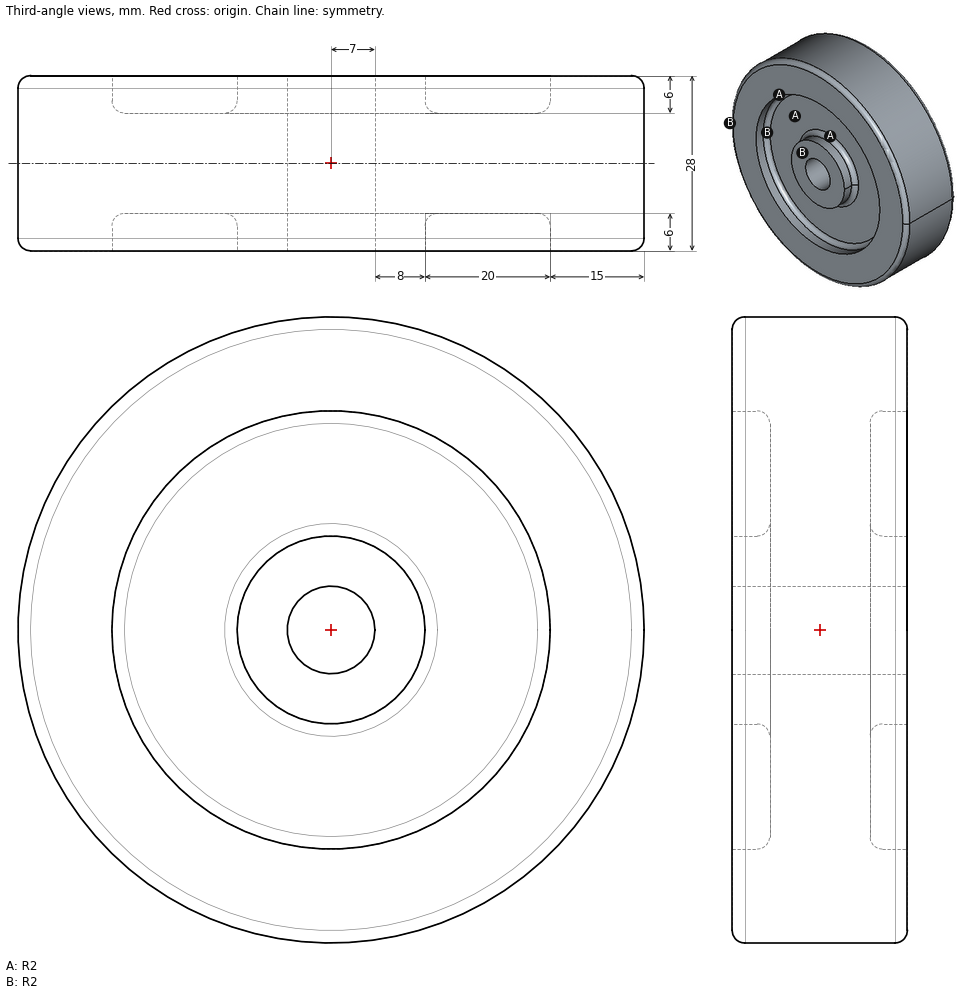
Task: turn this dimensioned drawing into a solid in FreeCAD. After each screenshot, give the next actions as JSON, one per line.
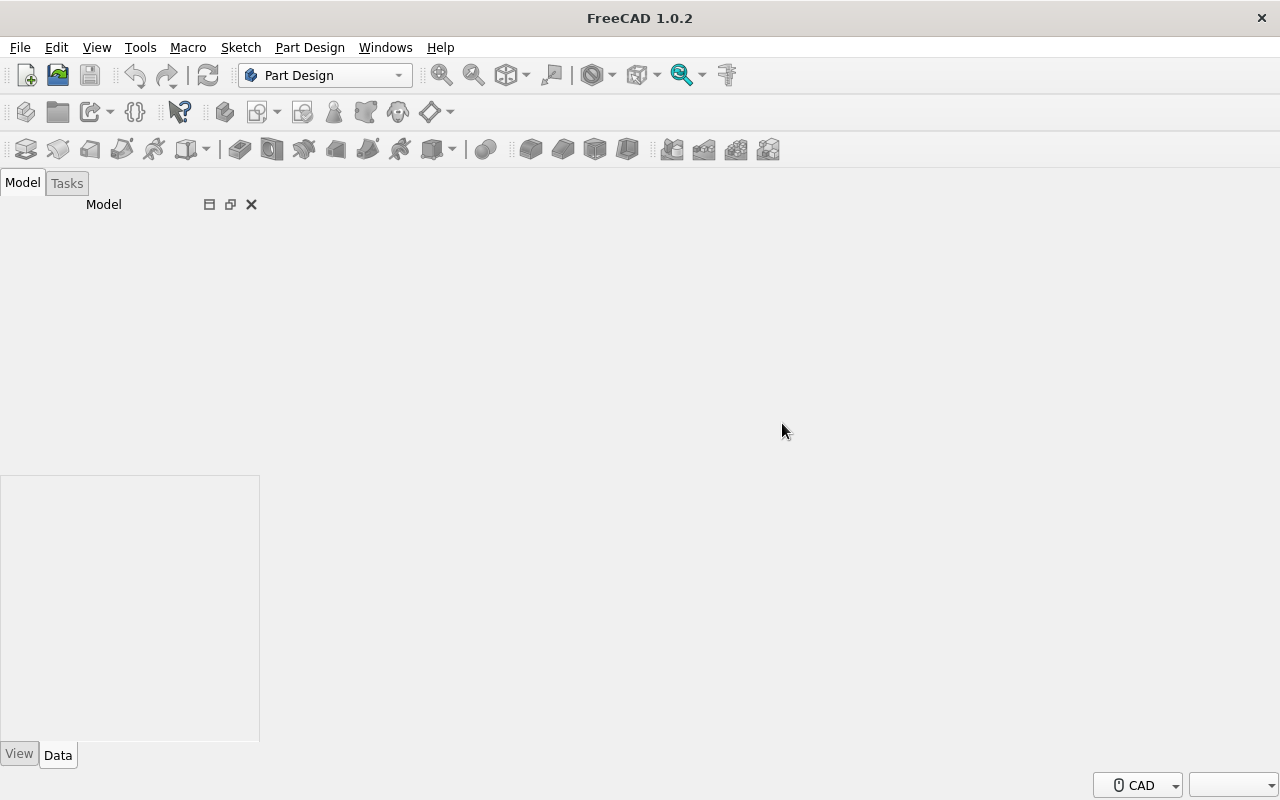
{"action": "left_click", "coordinate": [26, 76]}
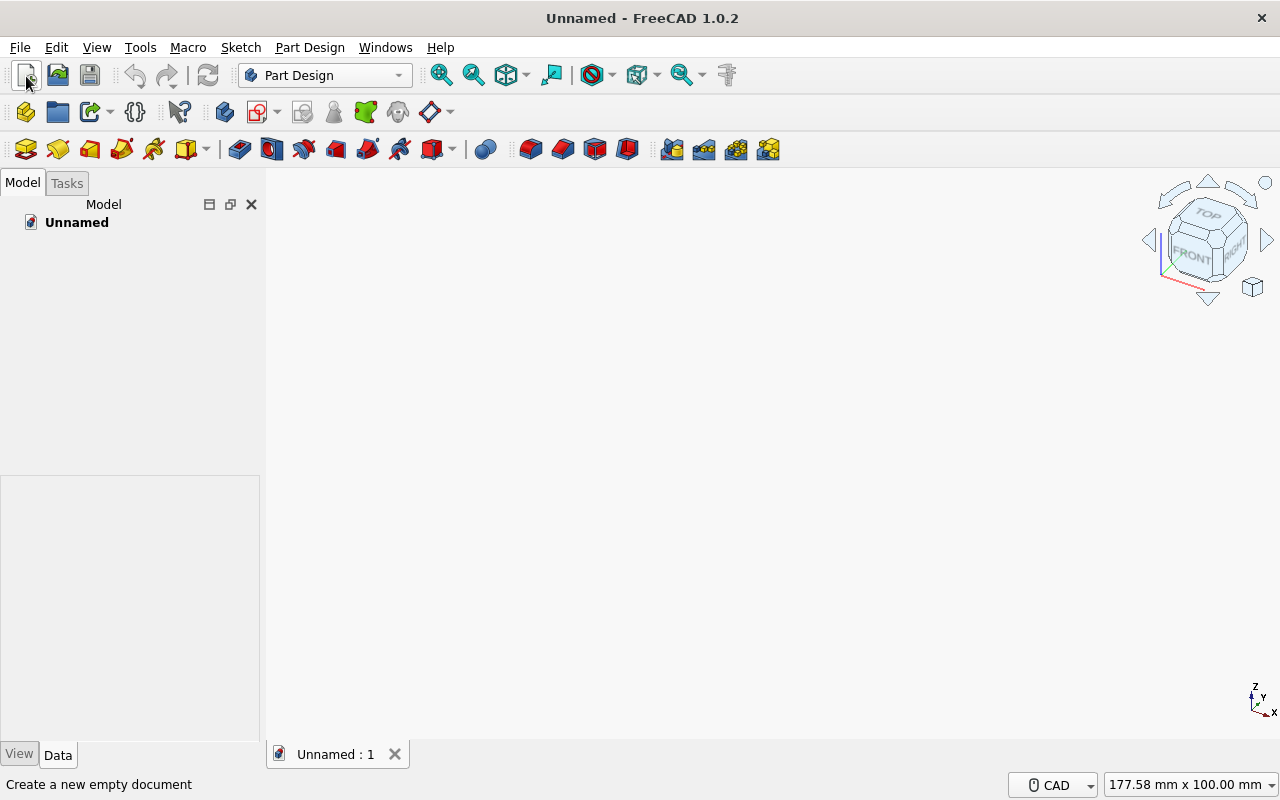
{"action": "left_click", "coordinate": [258, 112]}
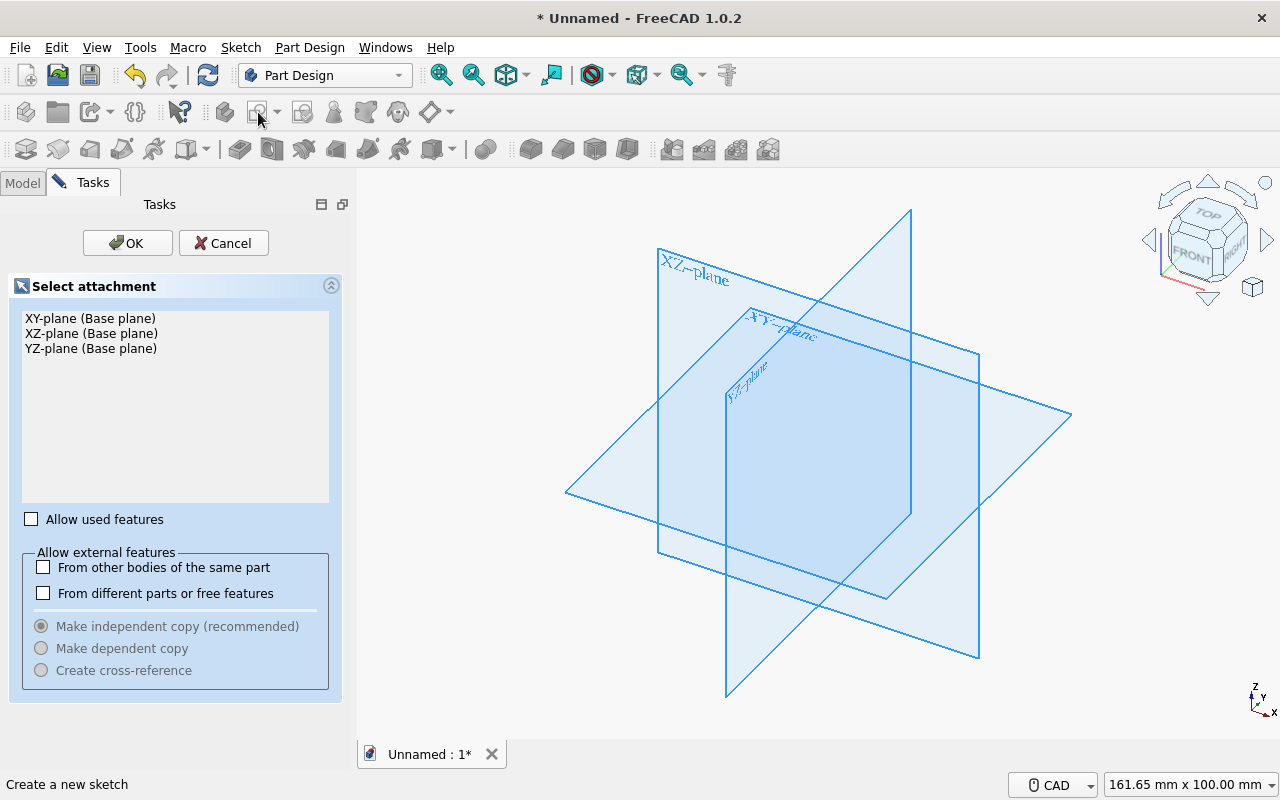
{"action": "left_click", "coordinate": [82, 318]}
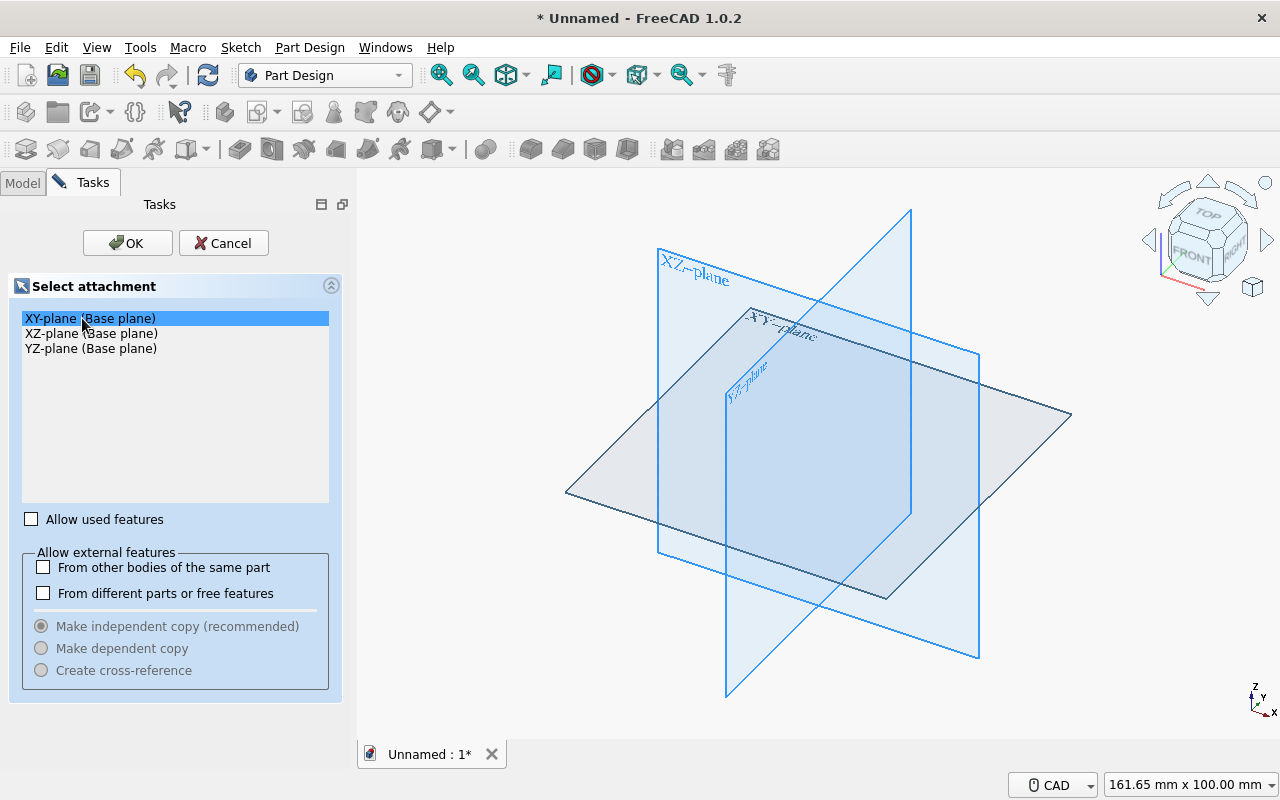
{"action": "left_click", "coordinate": [128, 243]}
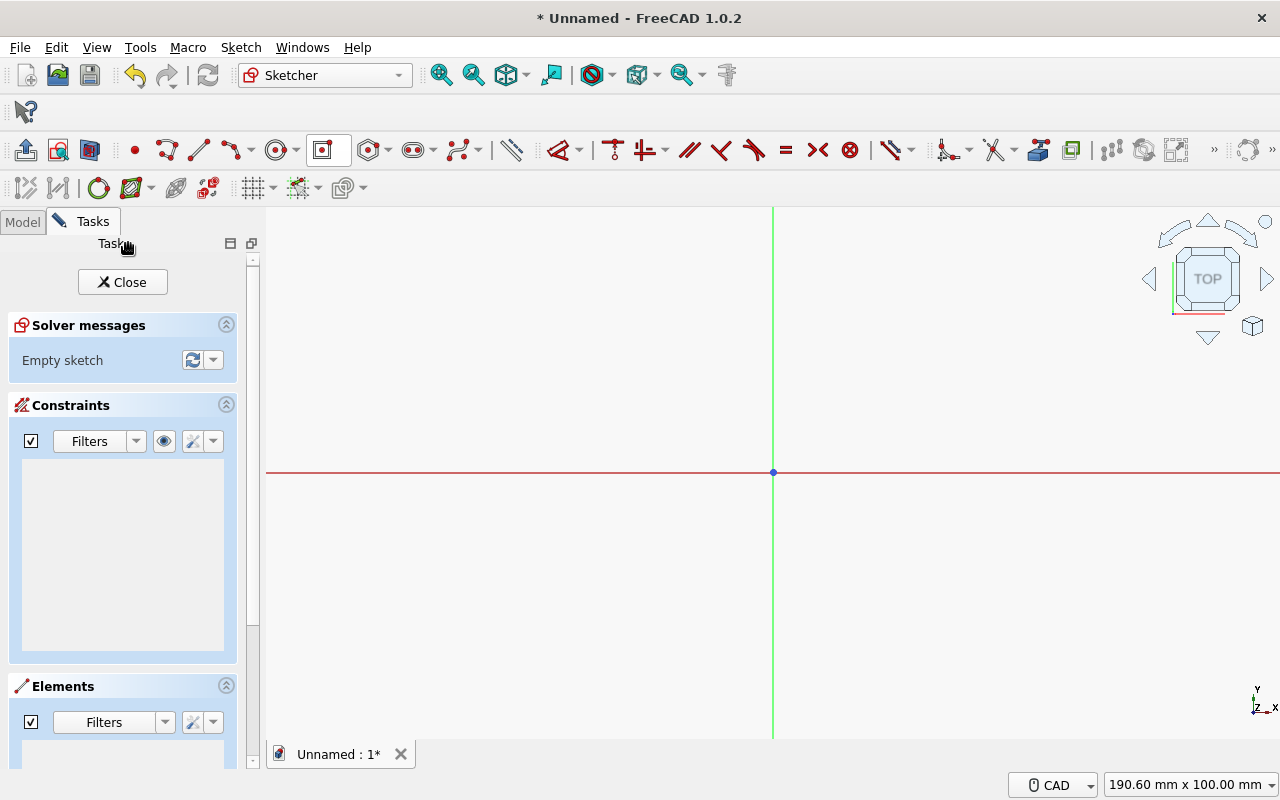
{"action": "scroll", "coordinate": [1070, 473], "scroll_direction": "up", "scroll_amount": 4}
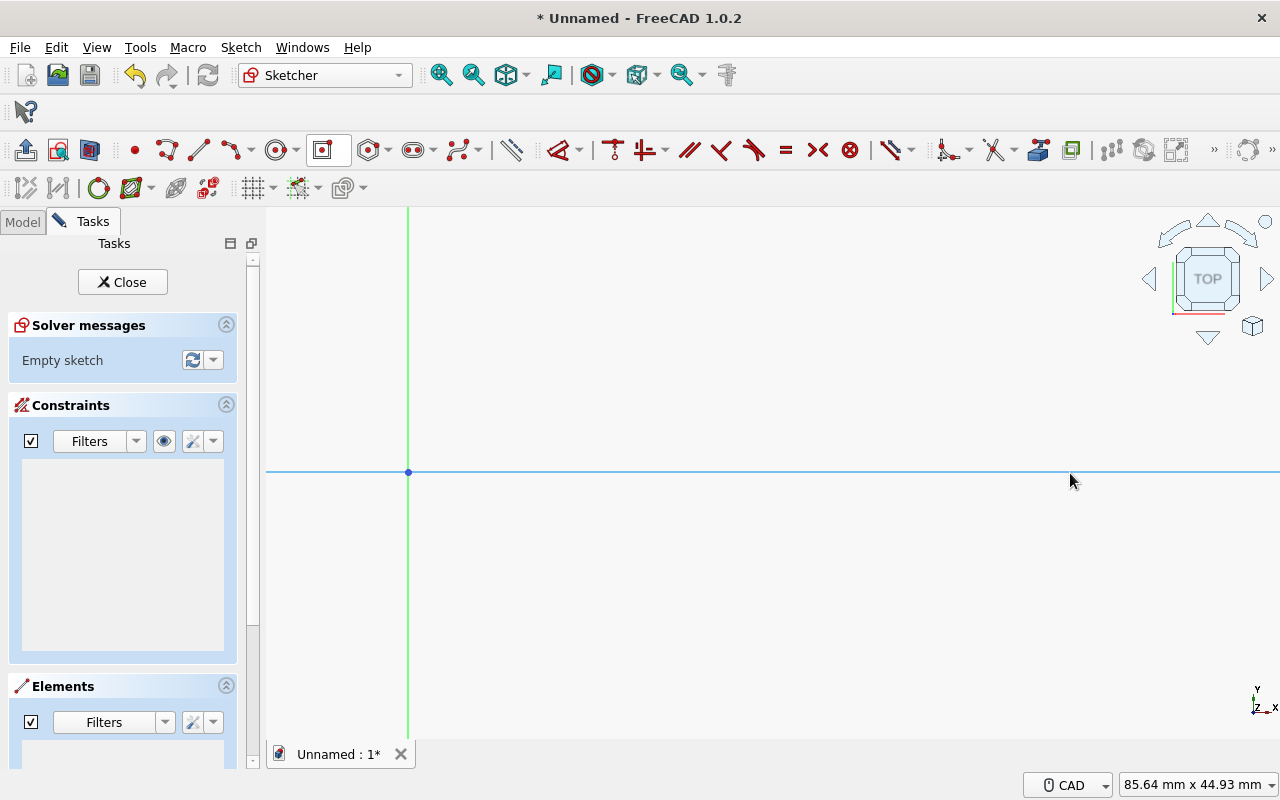
{"action": "left_click", "coordinate": [168, 150]}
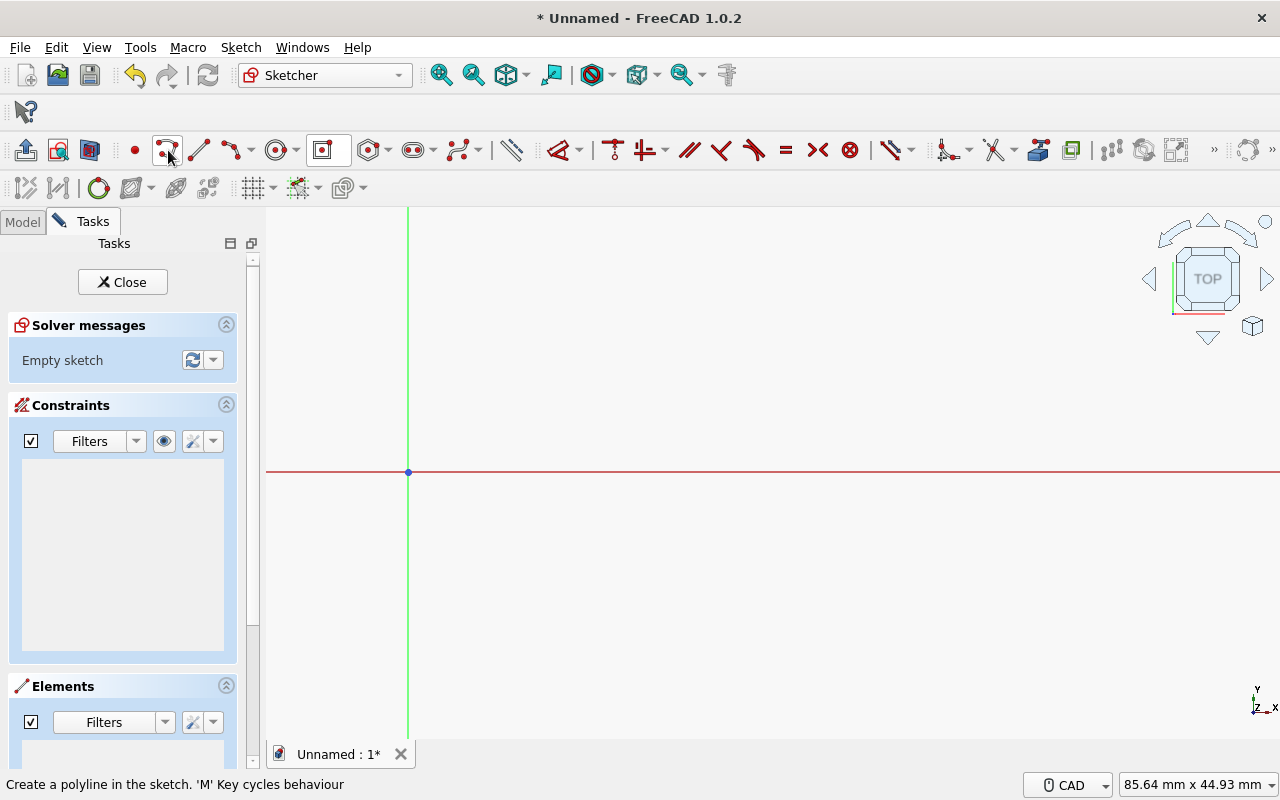
{"action": "left_click", "coordinate": [491, 307]}
{"action": "left_click", "coordinate": [491, 638]}
{"action": "left_click", "coordinate": [586, 638]}
{"action": "left_click", "coordinate": [586, 567]}
{"action": "left_click", "coordinate": [822, 567]}
{"action": "left_click", "coordinate": [822, 638]}
{"action": "left_click", "coordinate": [1000, 638]}
{"action": "left_click", "coordinate": [1000, 307]}
{"action": "left_click", "coordinate": [822, 307]}
{"action": "left_click", "coordinate": [822, 378]}
{"action": "left_click", "coordinate": [586, 378]}
{"action": "left_click", "coordinate": [586, 307]}
{"action": "left_click", "coordinate": [491, 308]}
{"action": "key", "text": "Escape"}
{"action": "key", "text": "Escape"}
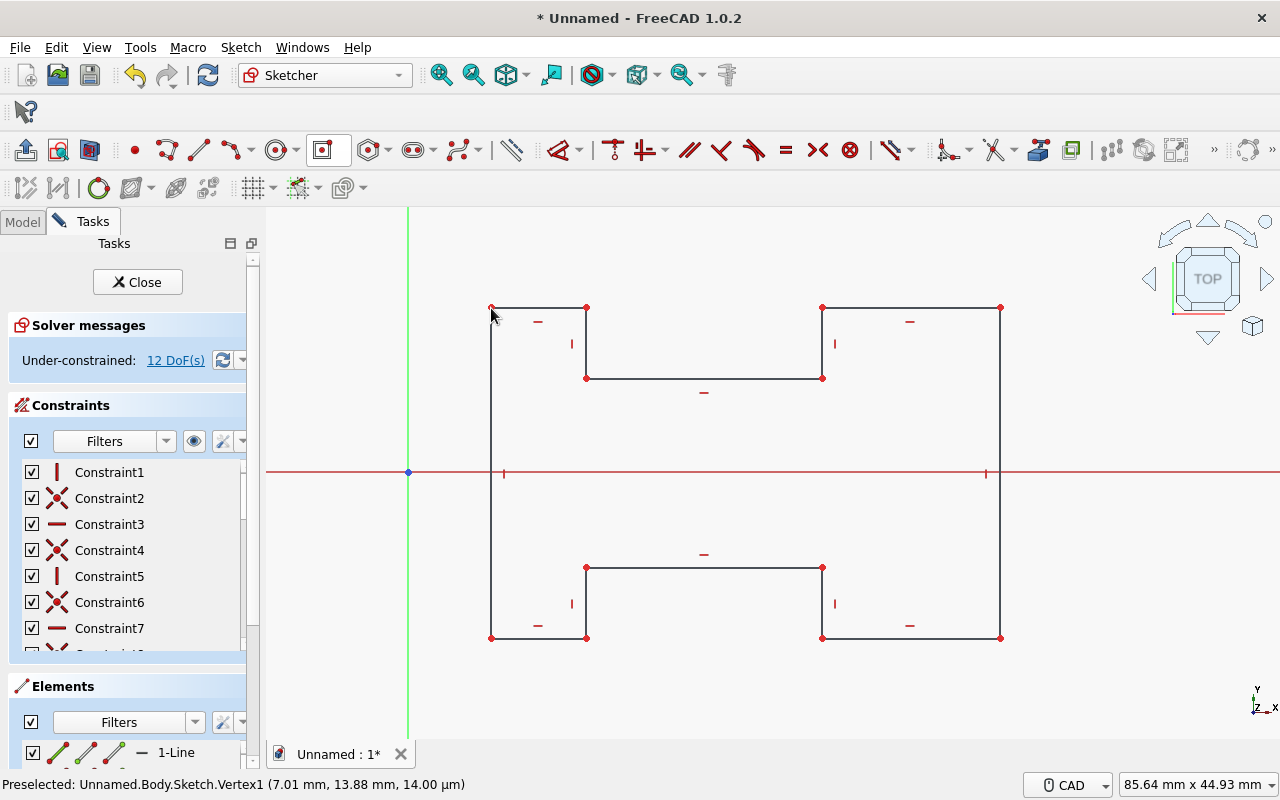
{"action": "left_click", "coordinate": [822, 639]}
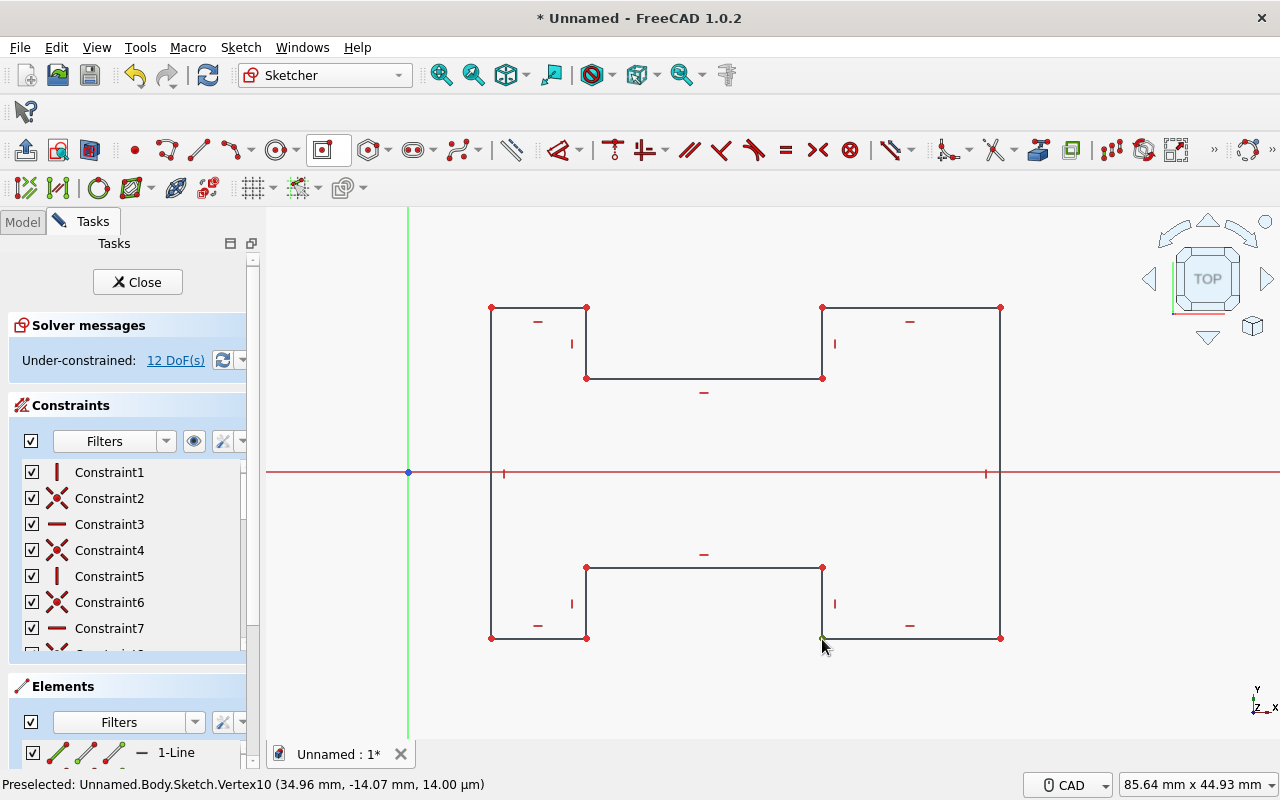
{"action": "left_click", "coordinate": [822, 308]}